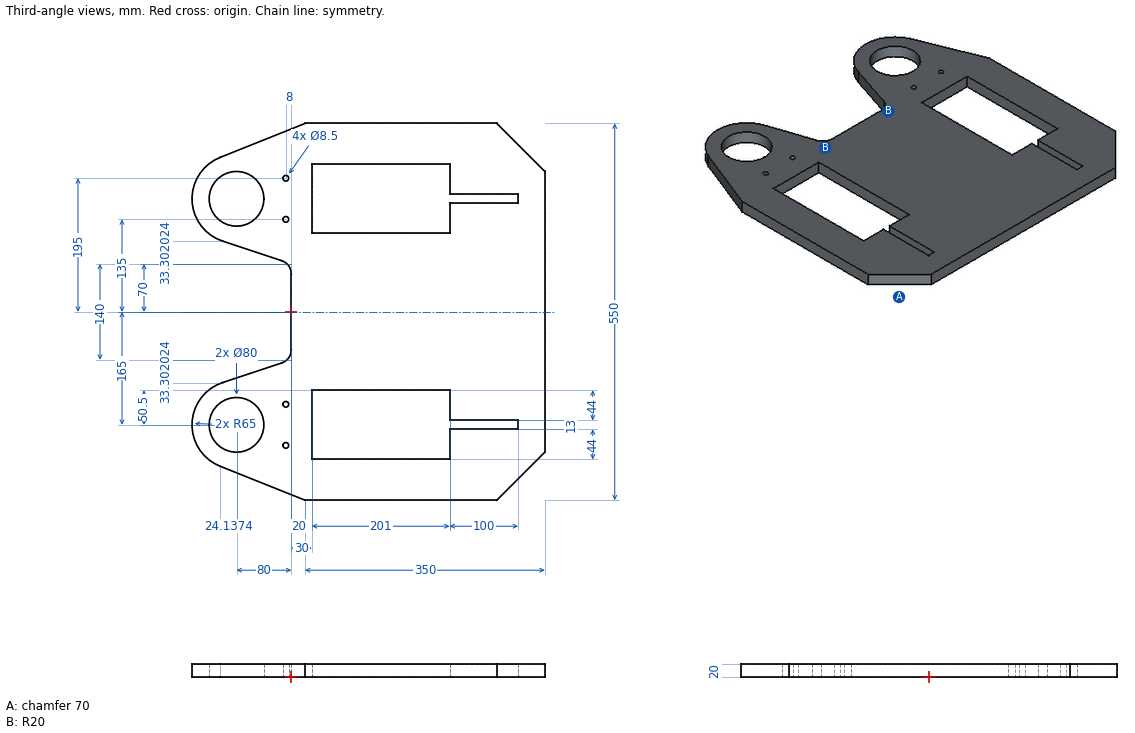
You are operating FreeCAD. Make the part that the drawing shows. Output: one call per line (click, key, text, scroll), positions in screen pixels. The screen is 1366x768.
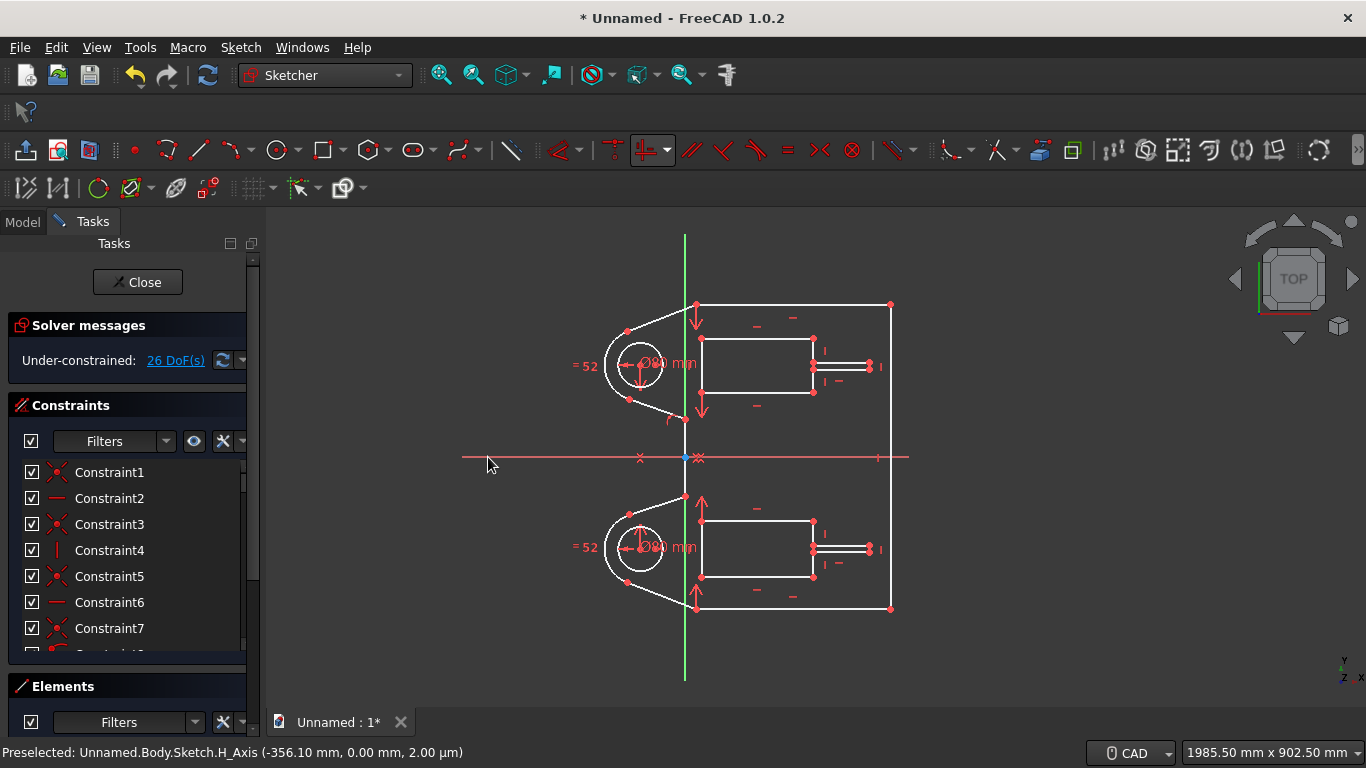
click(813, 577)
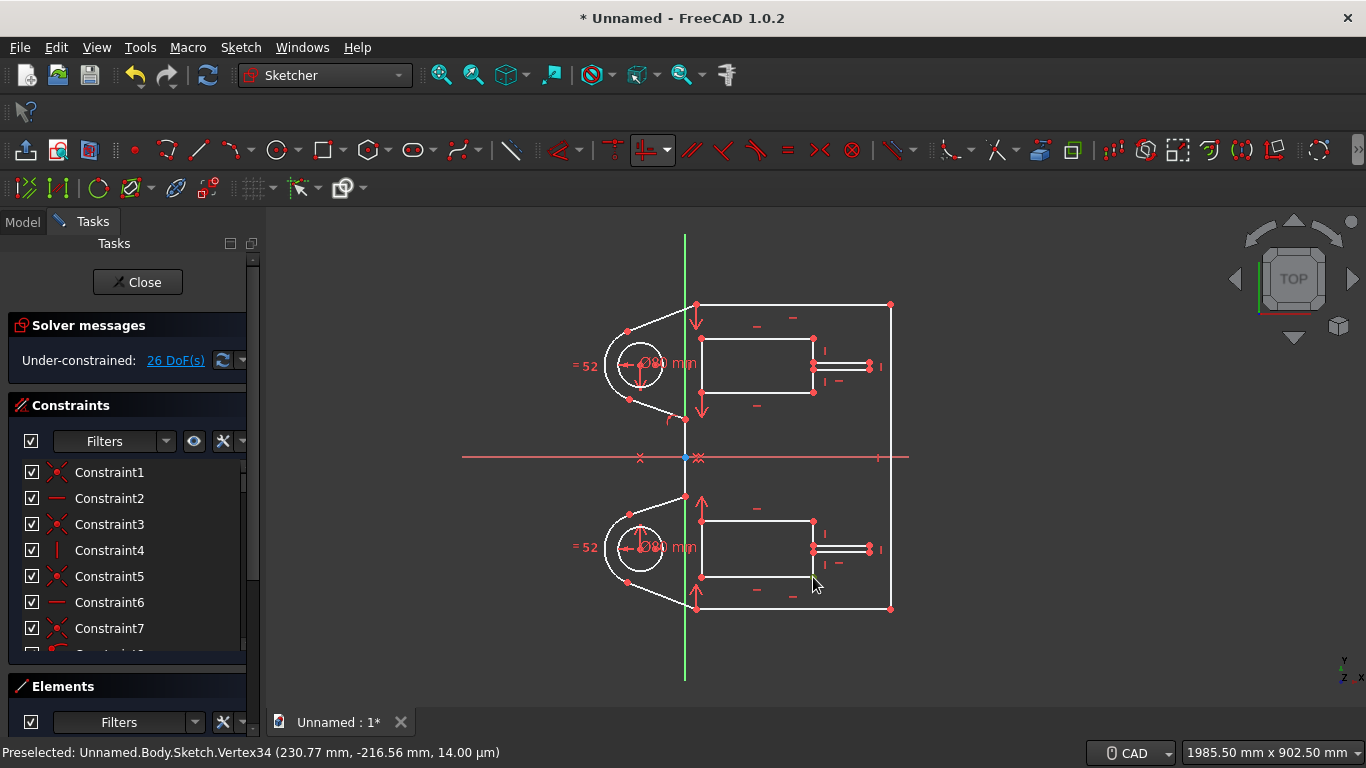
click(813, 339)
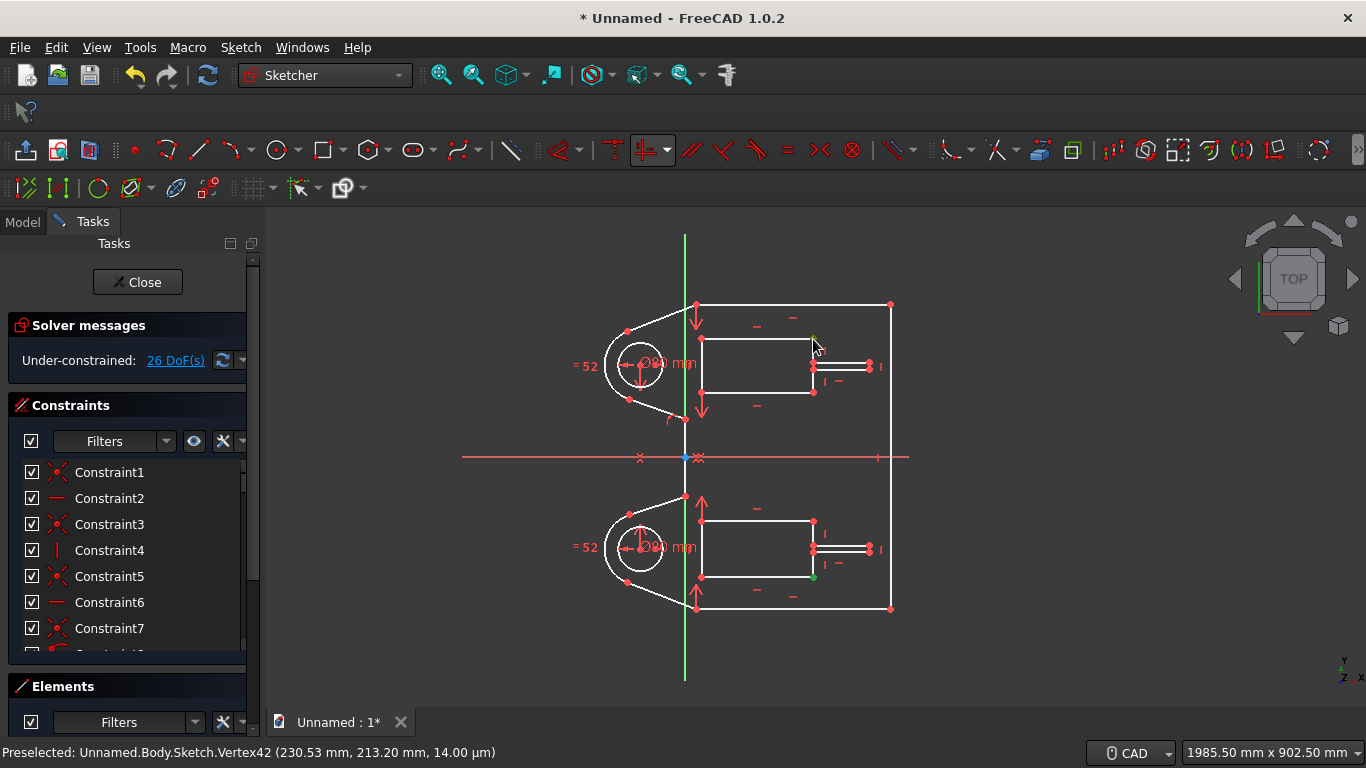
click(488, 457)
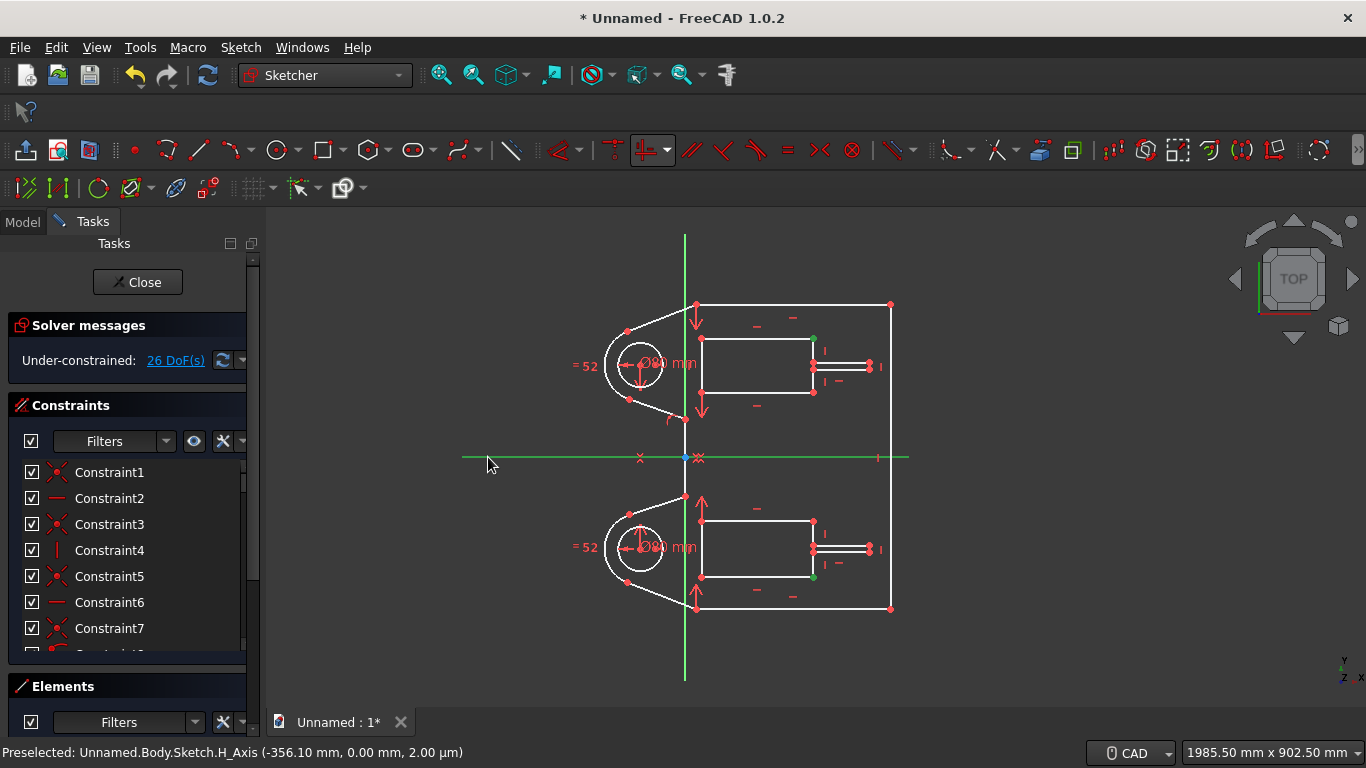
key(s)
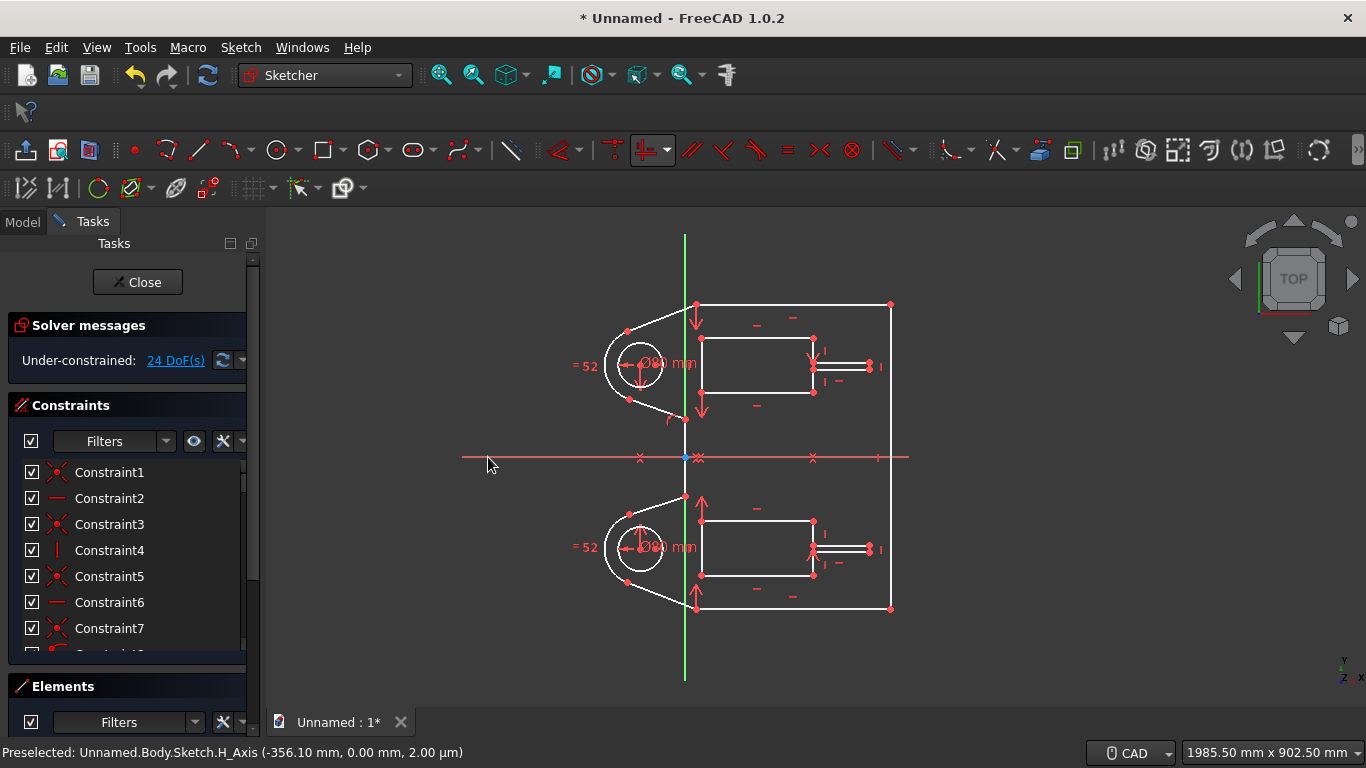
scroll(869, 552, up, 4)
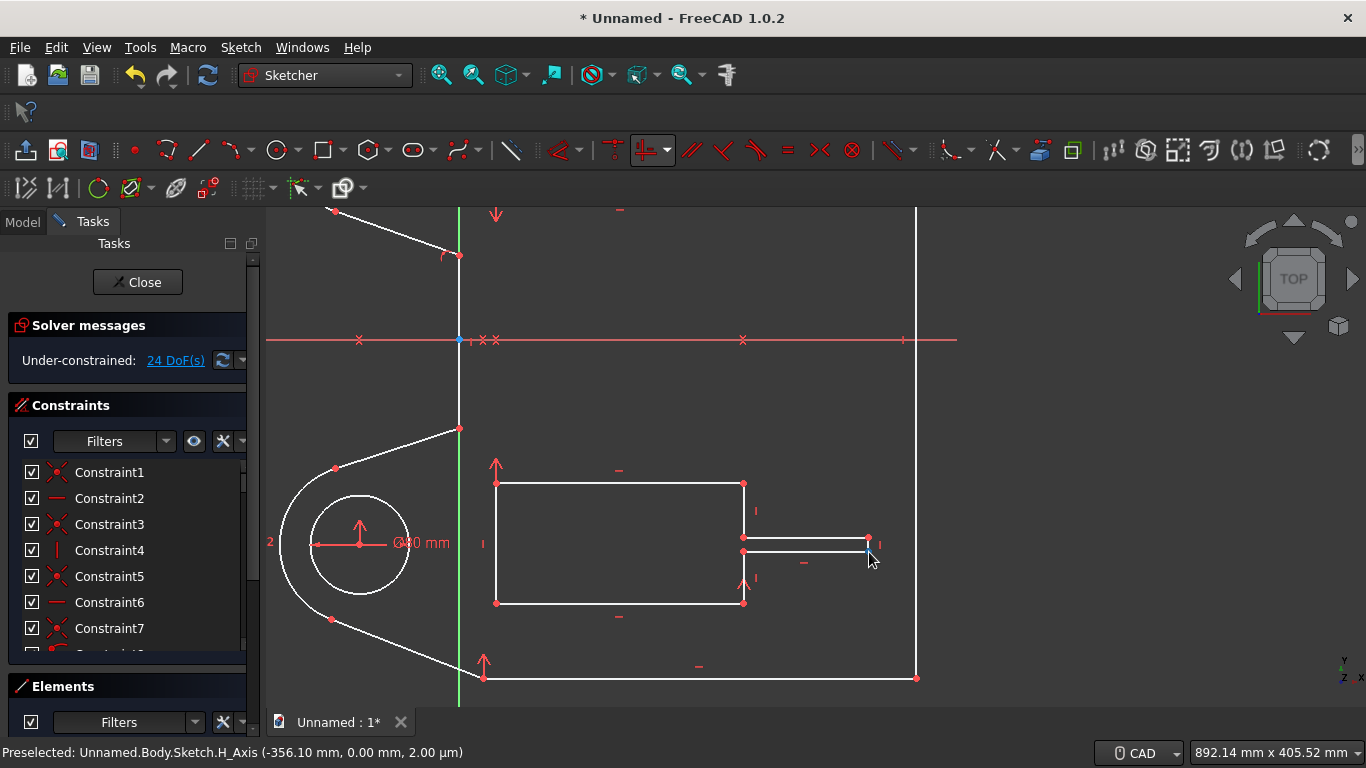
click(868, 552)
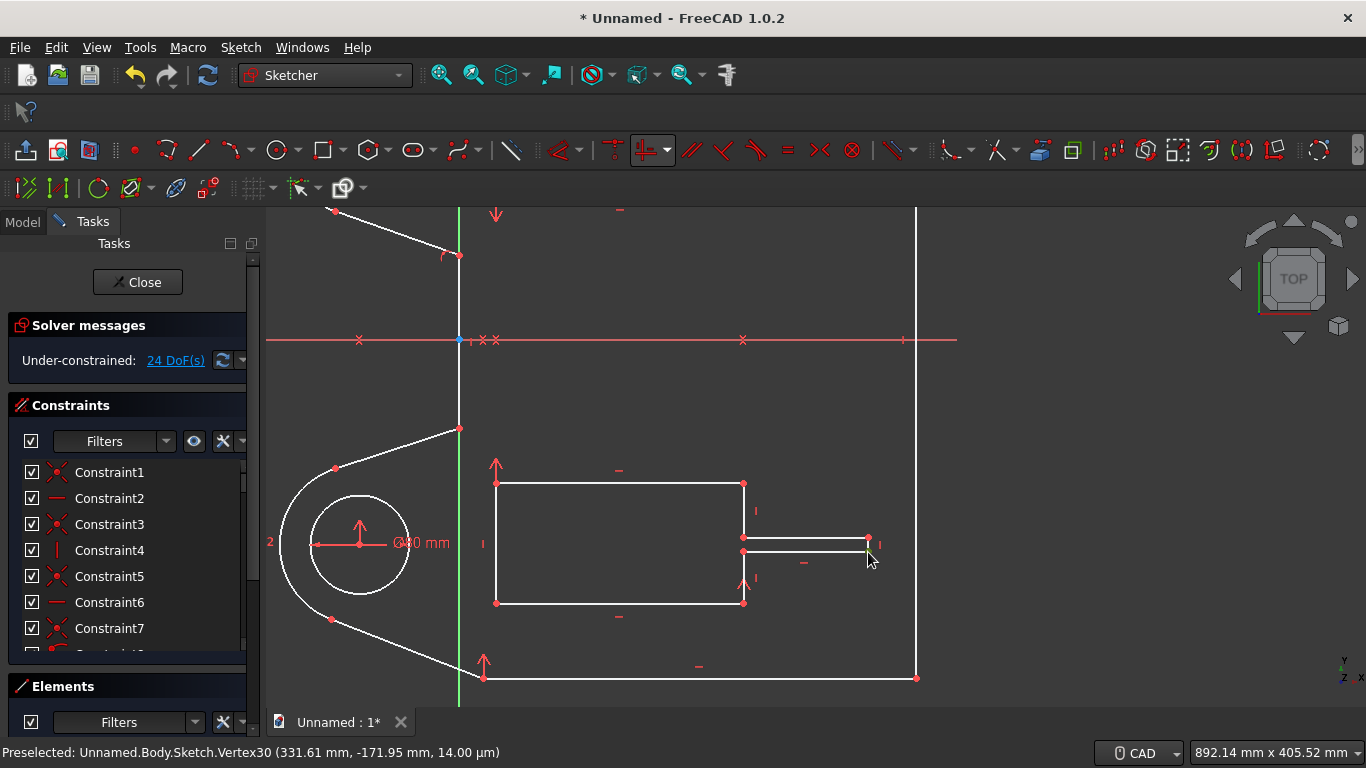
scroll(869, 552, down, 4)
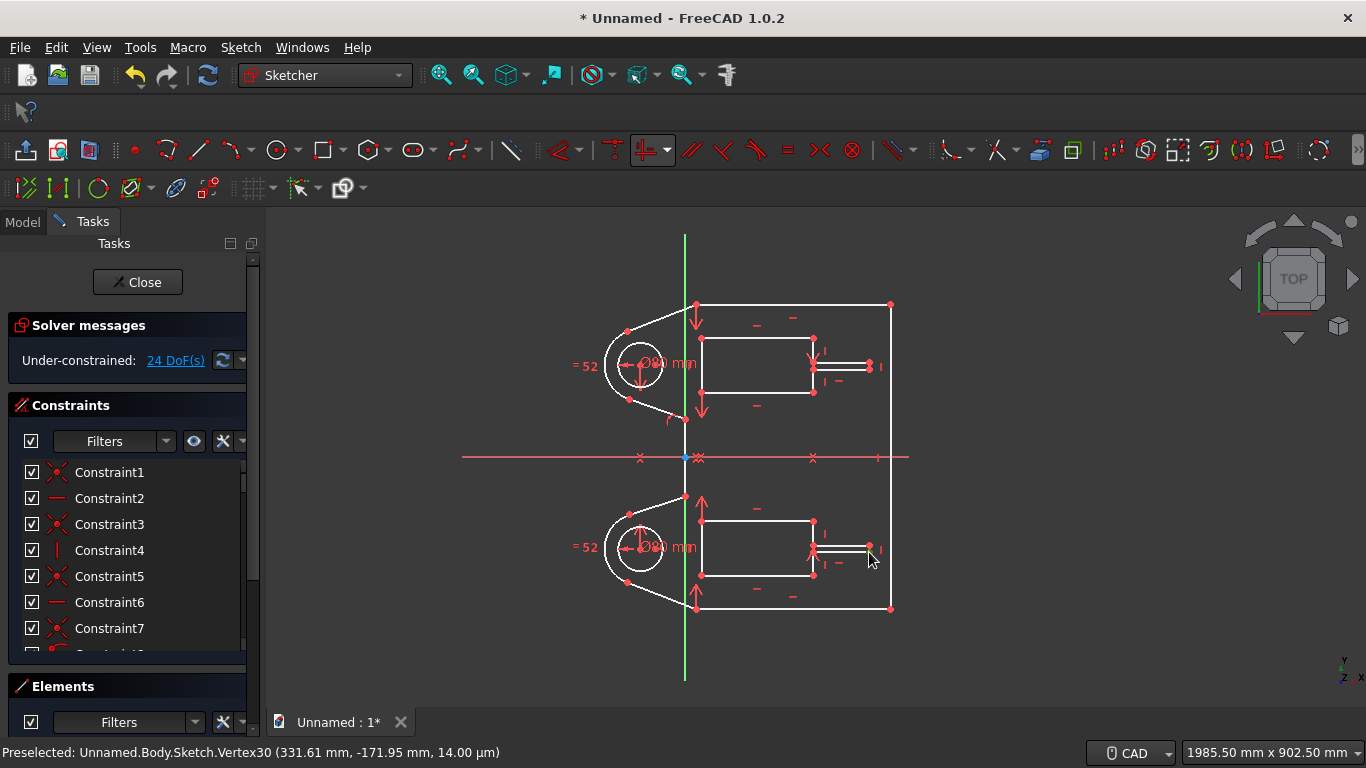
scroll(869, 363, up, 4)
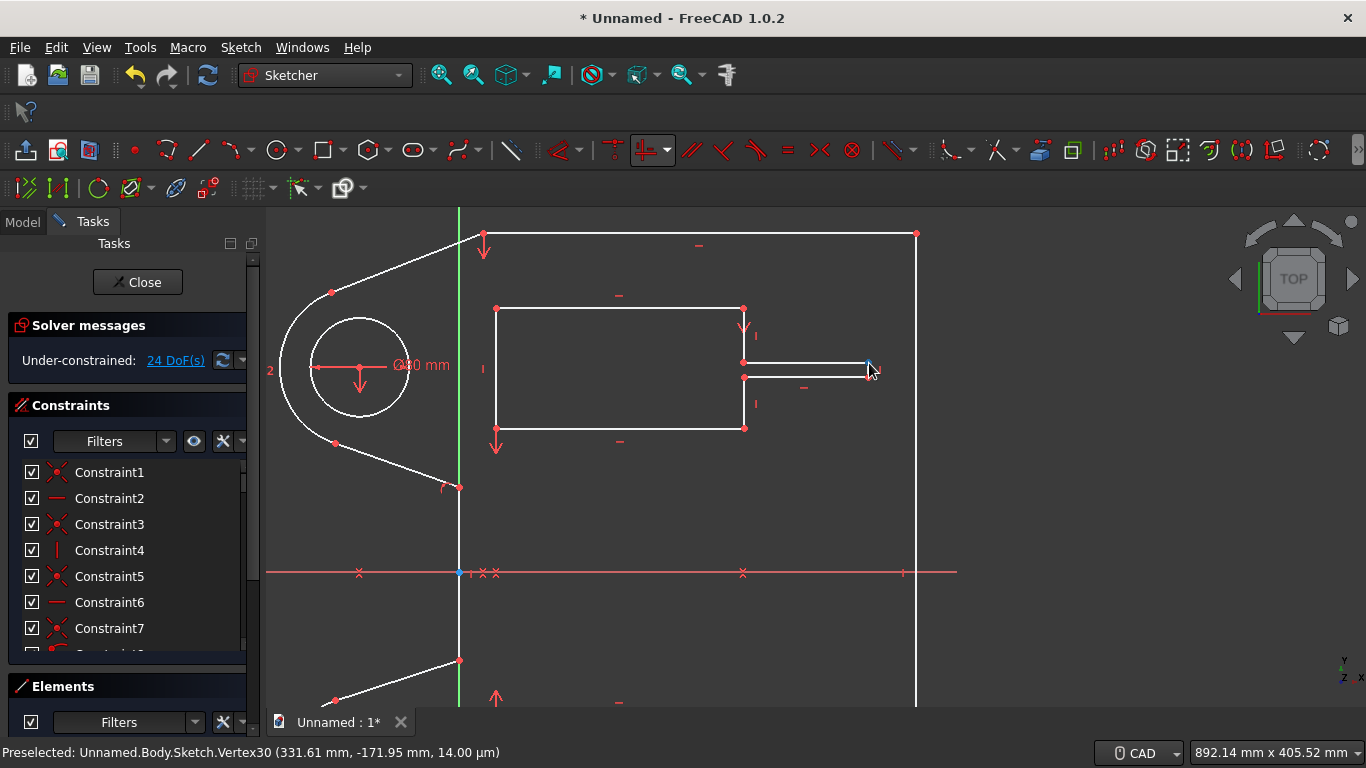
click(868, 363)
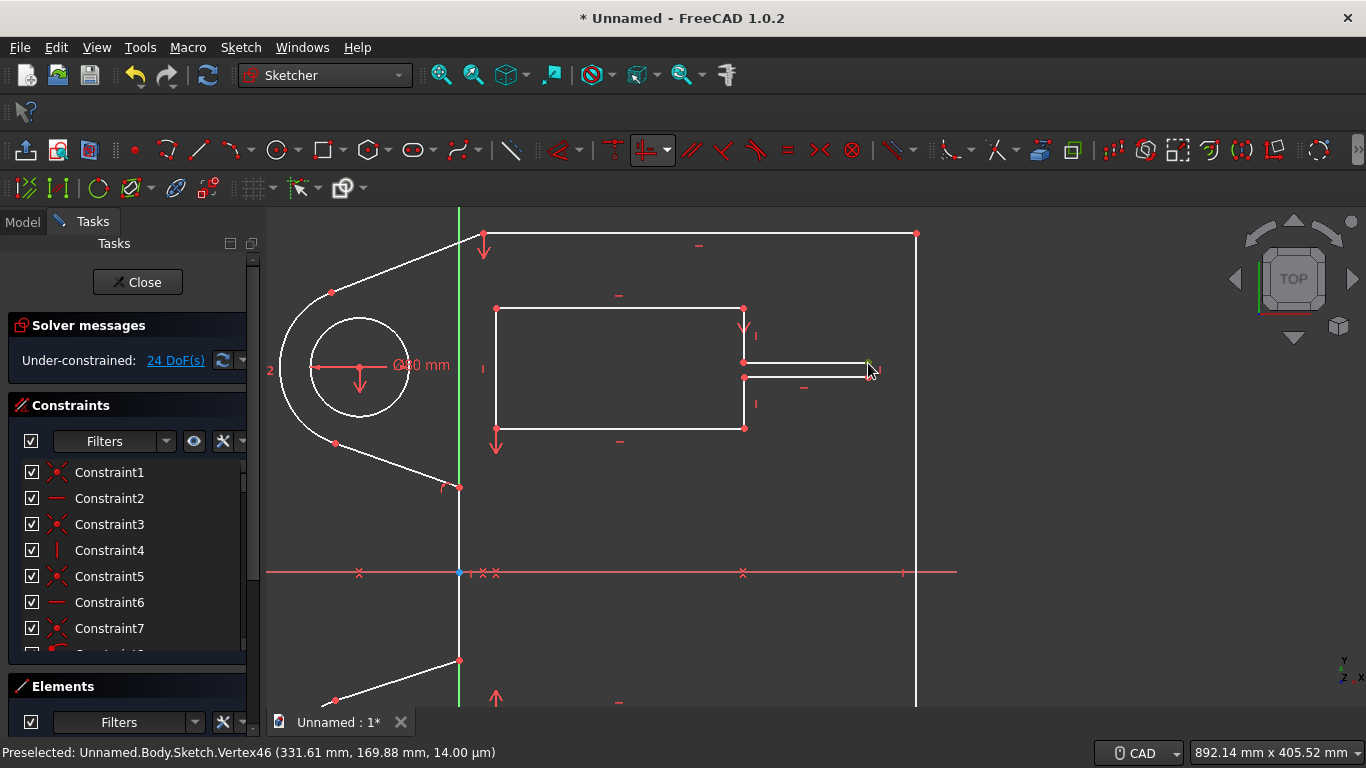
click(424, 572)